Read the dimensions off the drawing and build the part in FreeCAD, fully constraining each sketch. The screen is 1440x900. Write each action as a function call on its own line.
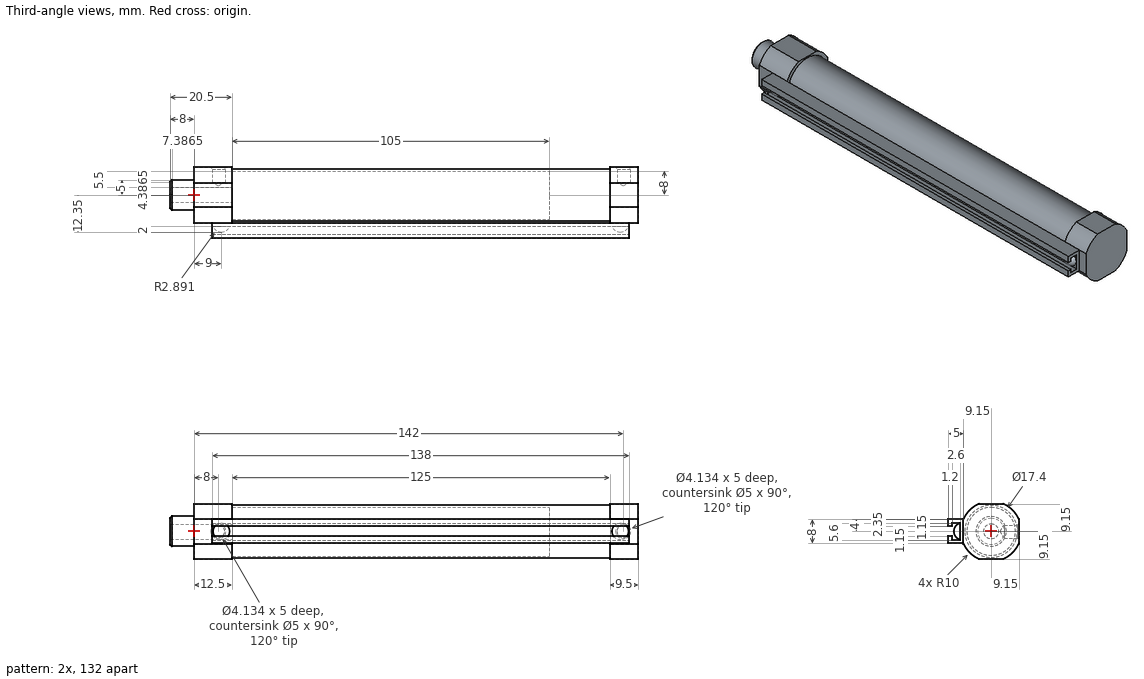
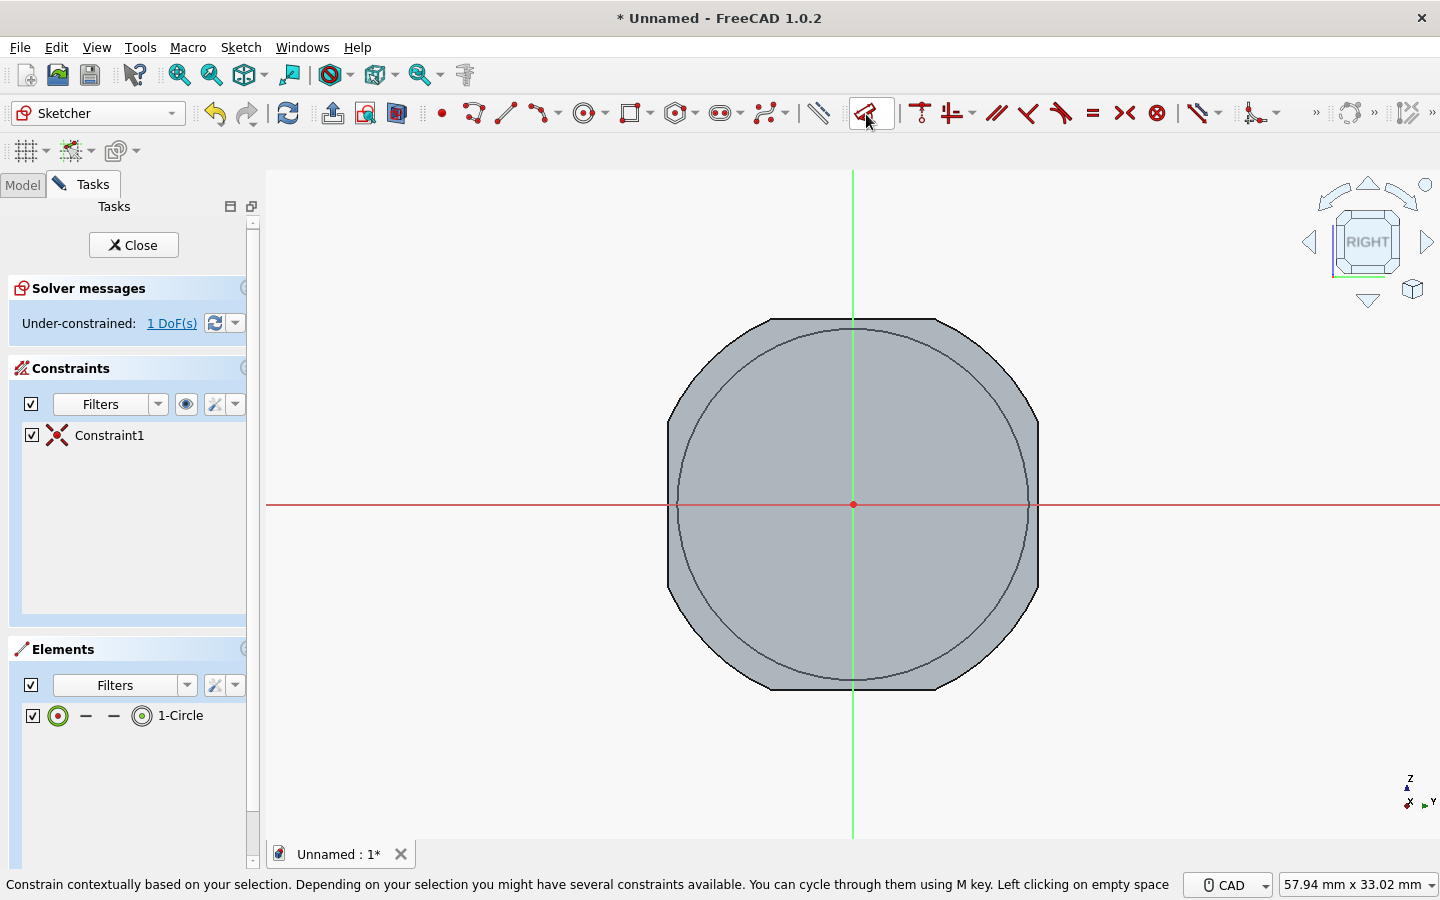
click(977, 380)
click(1000, 357)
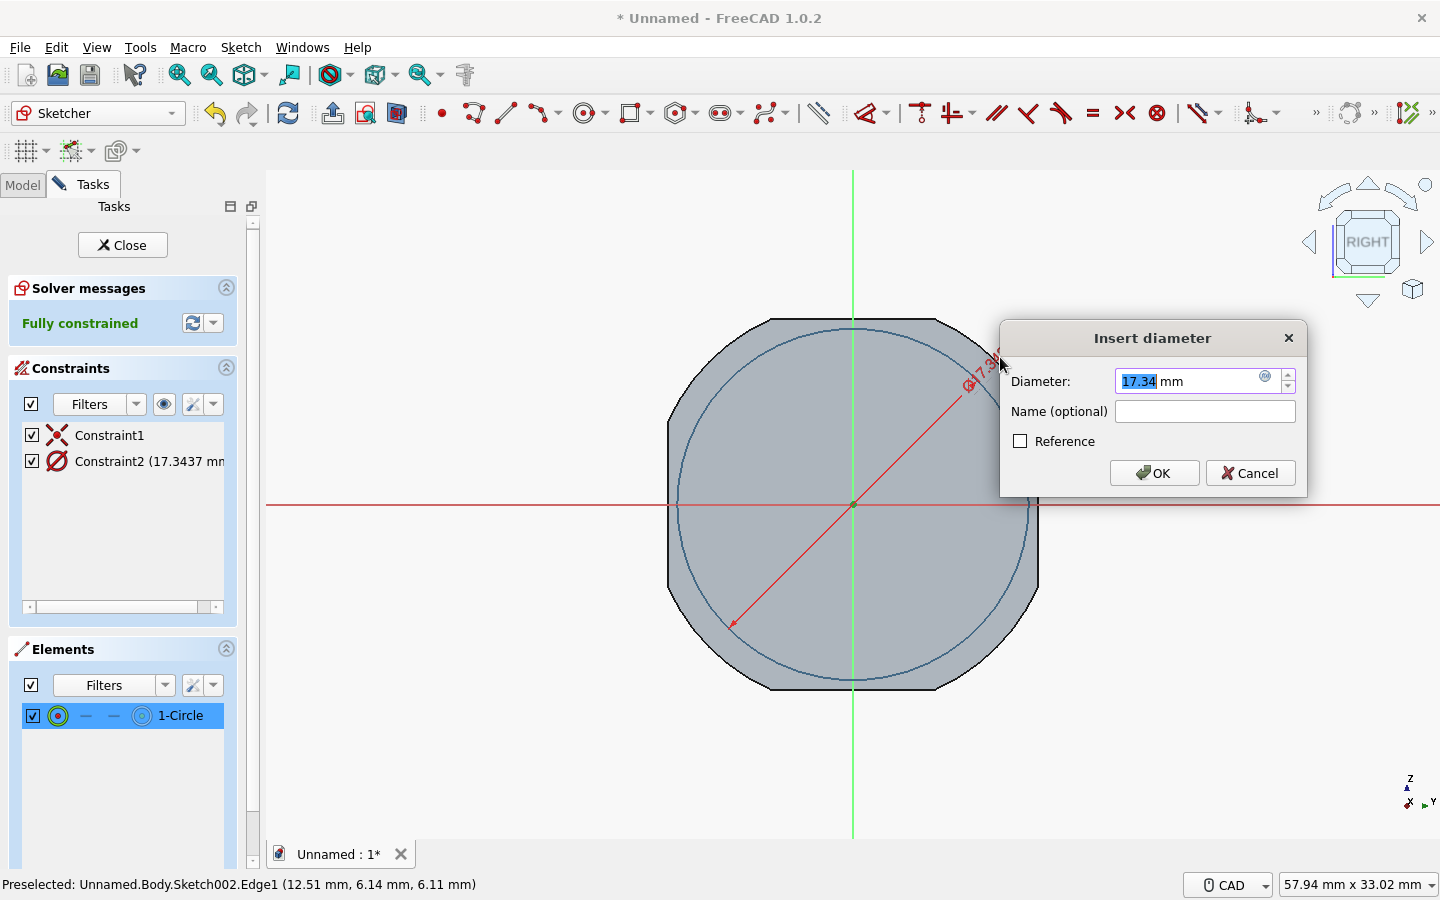
text(17.4)
key(Return)
key(Escape)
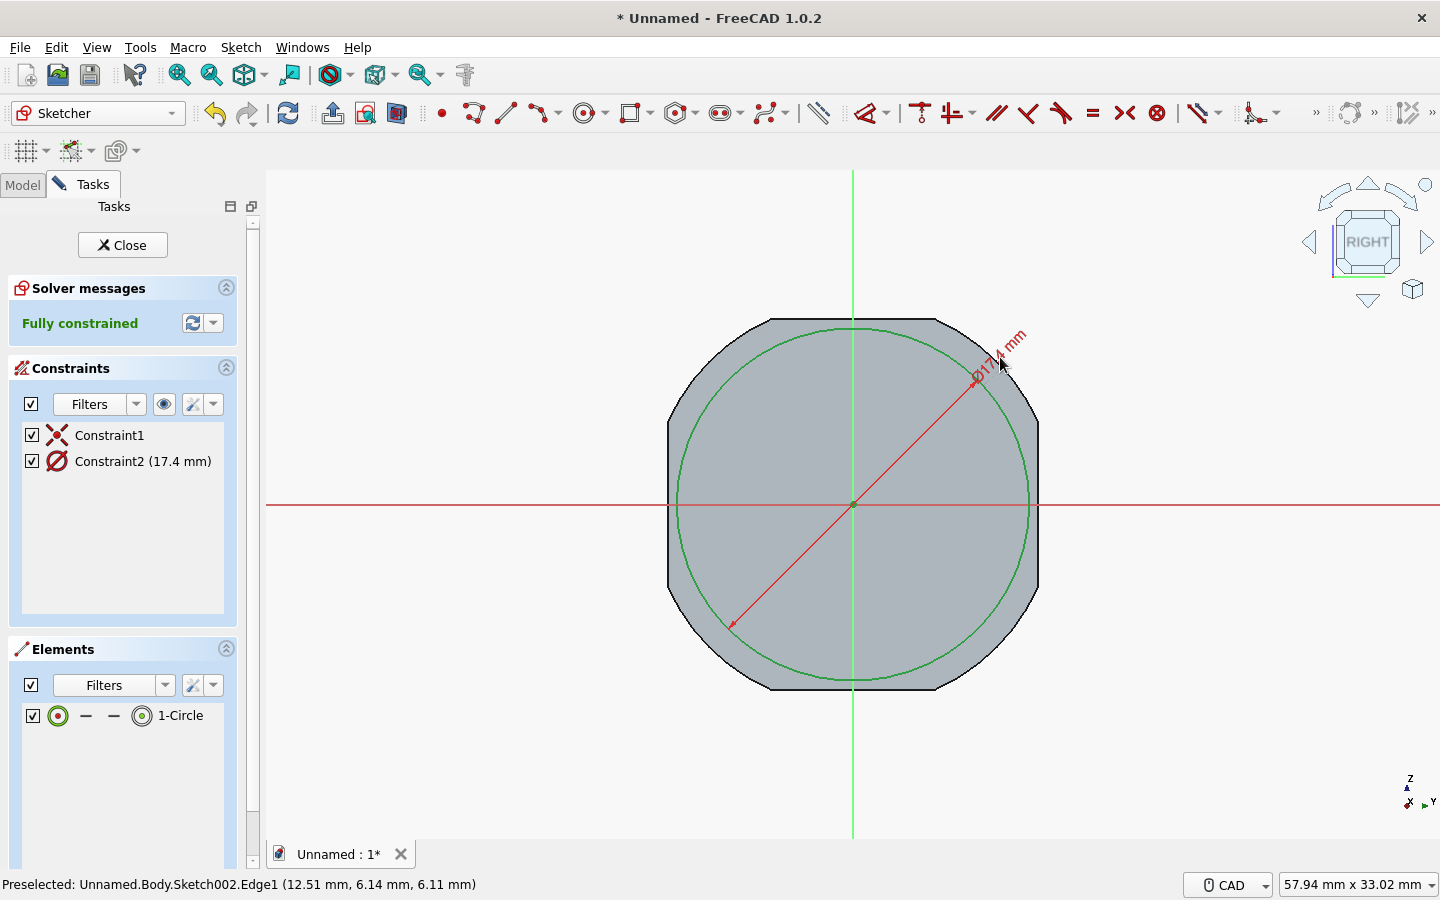
click(123, 245)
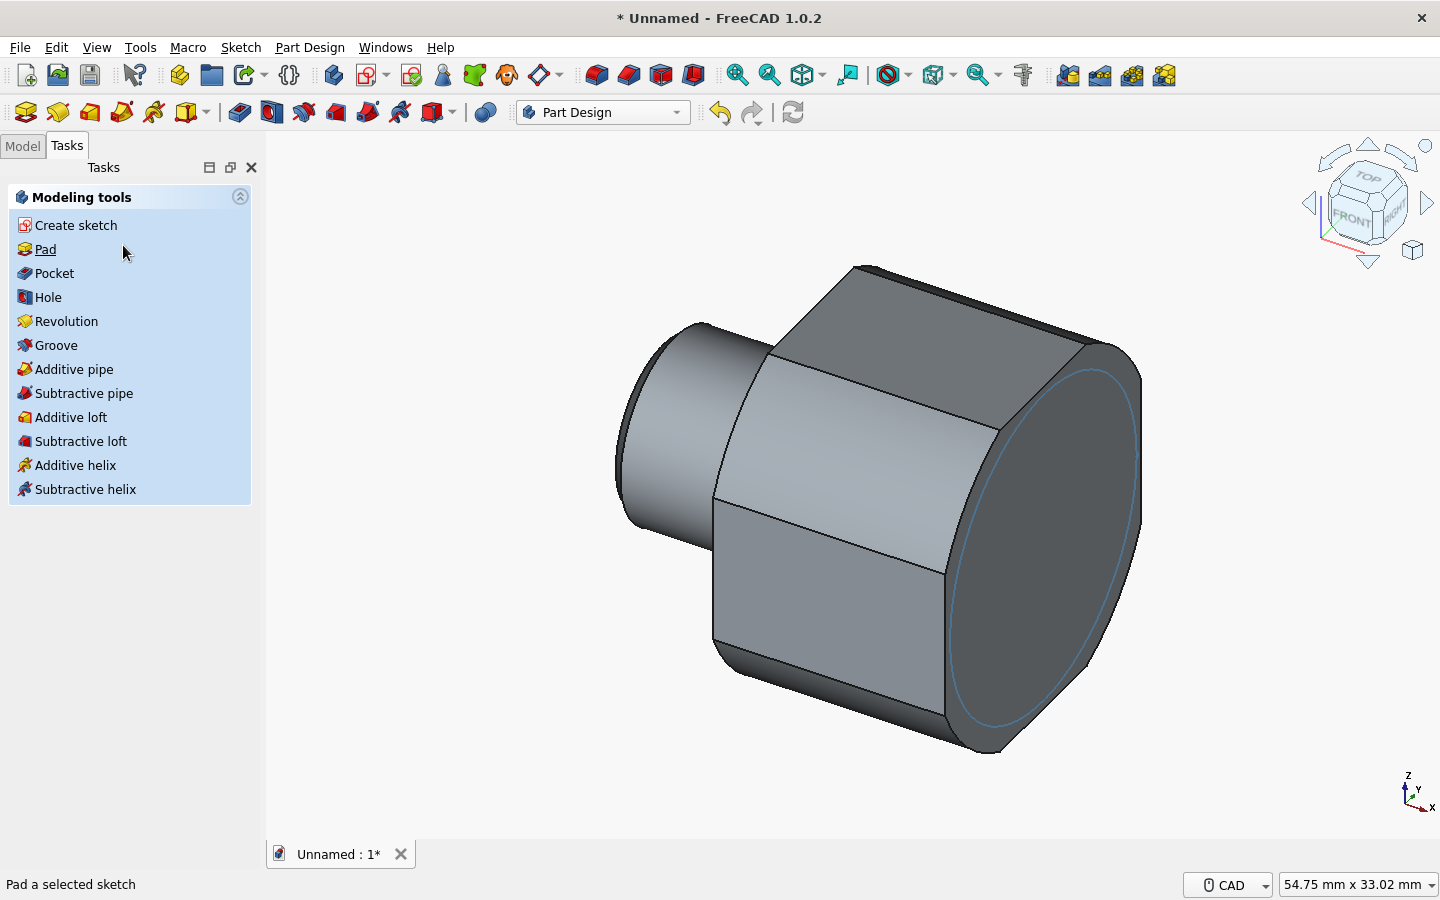
click(26, 112)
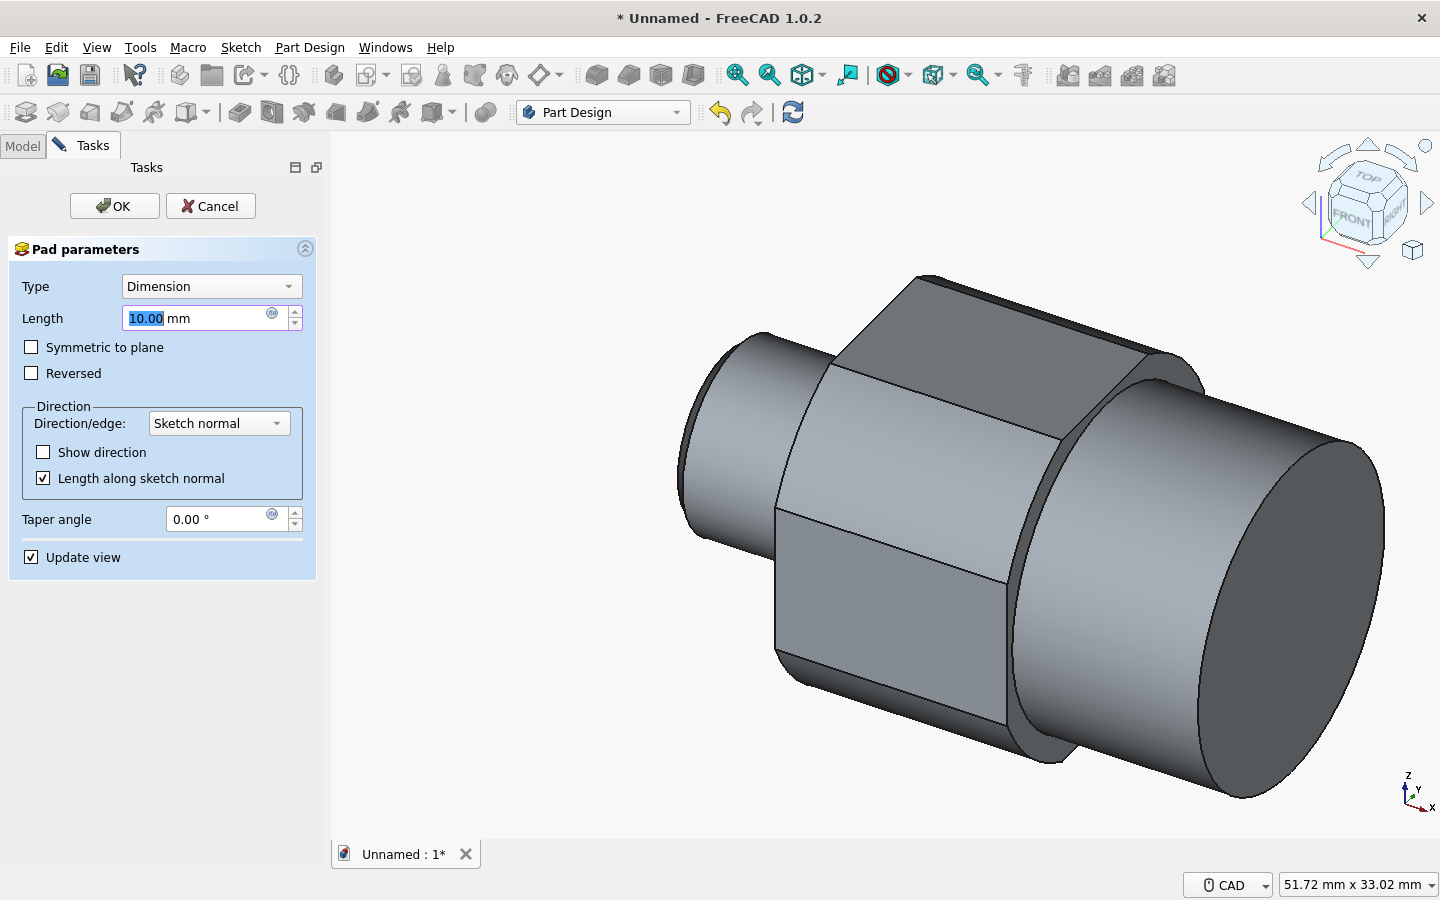
text(125)
key(Tab)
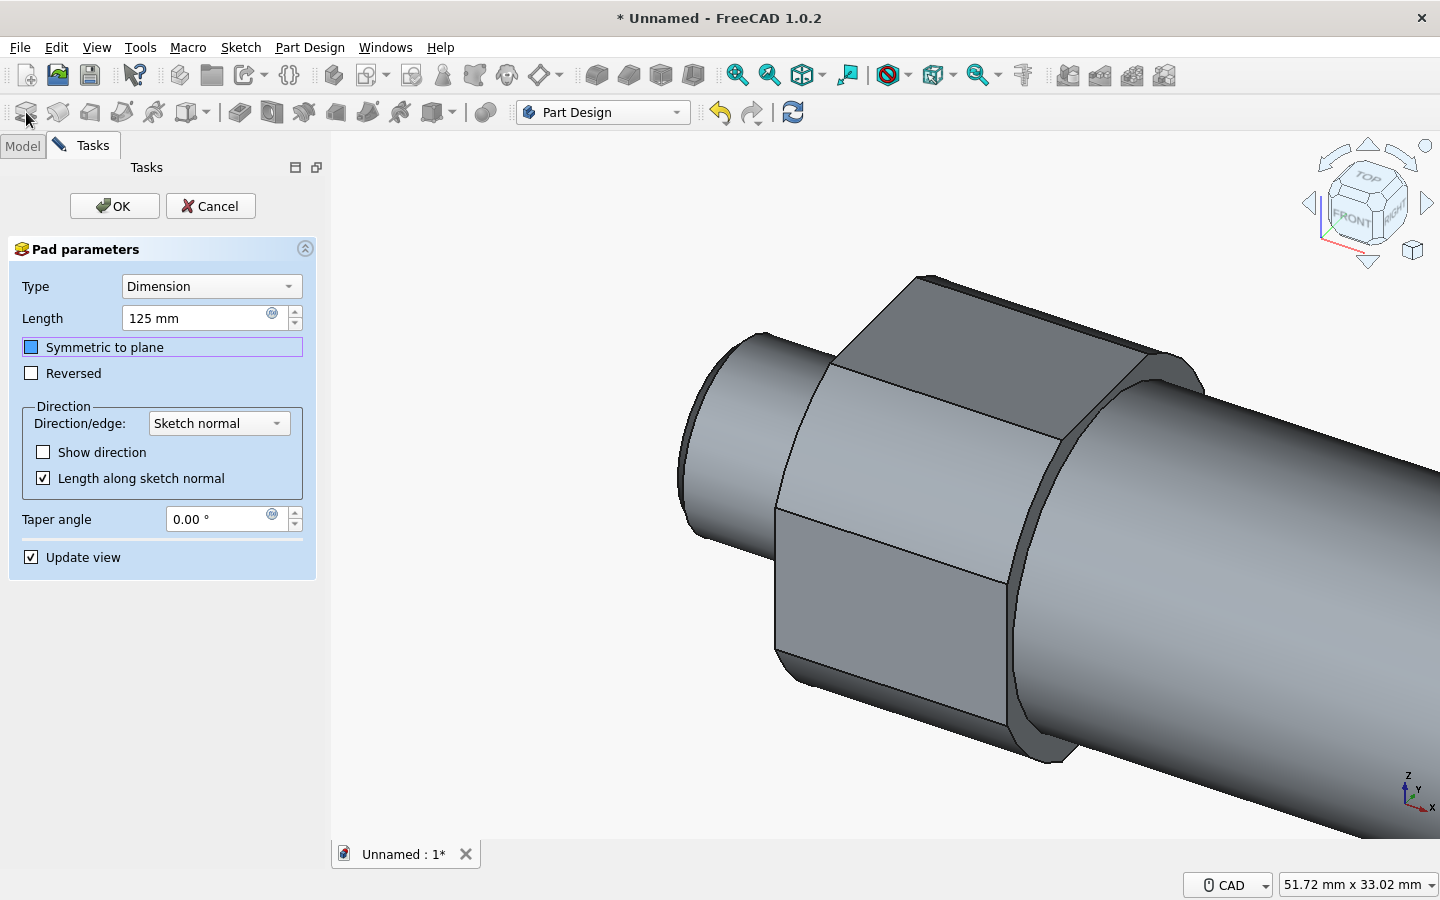
click(115, 206)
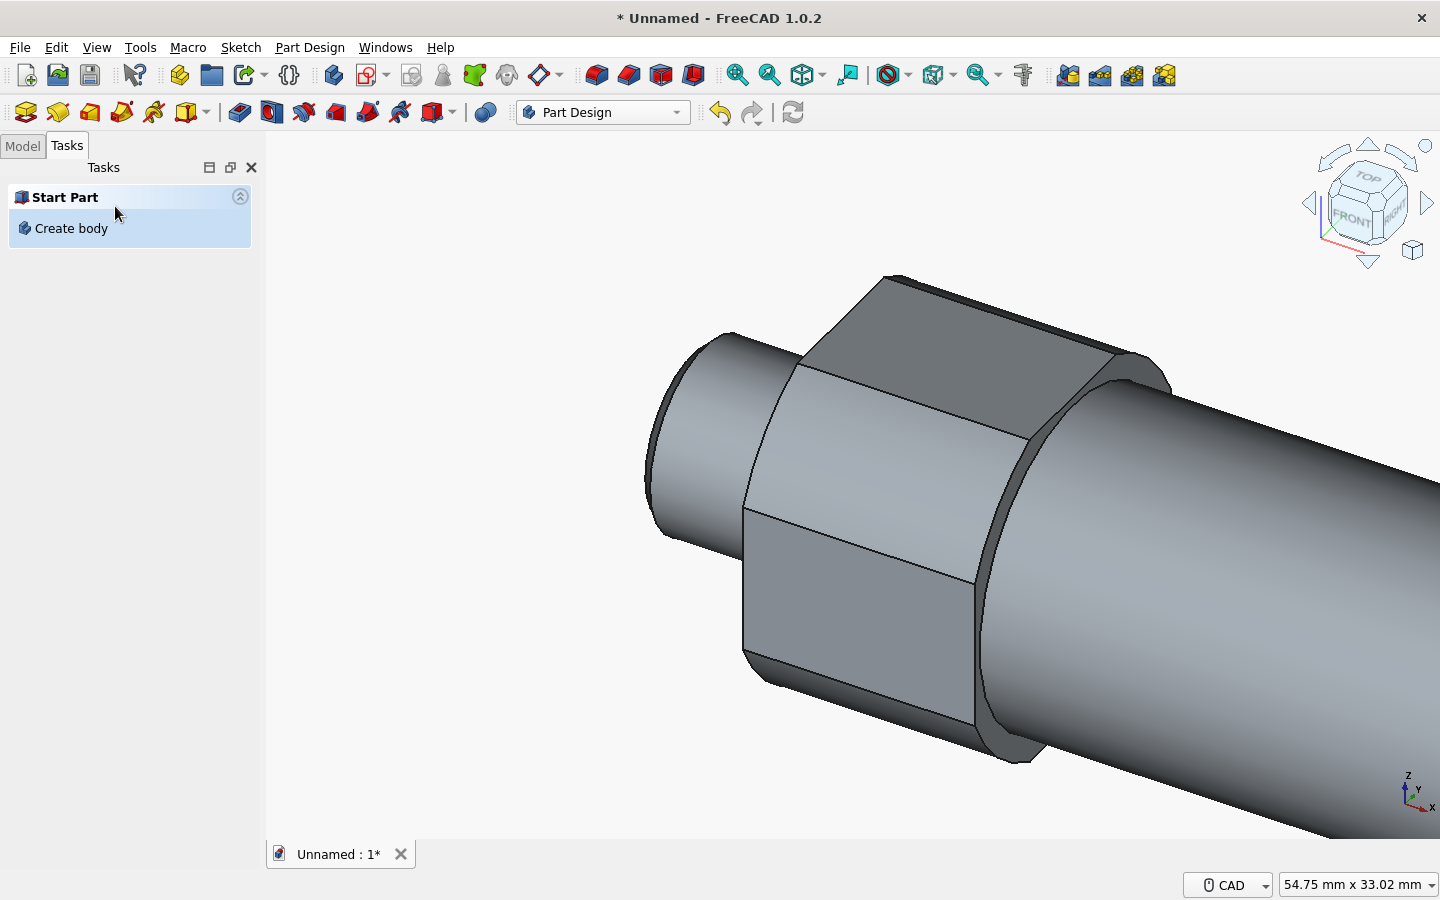
click(738, 76)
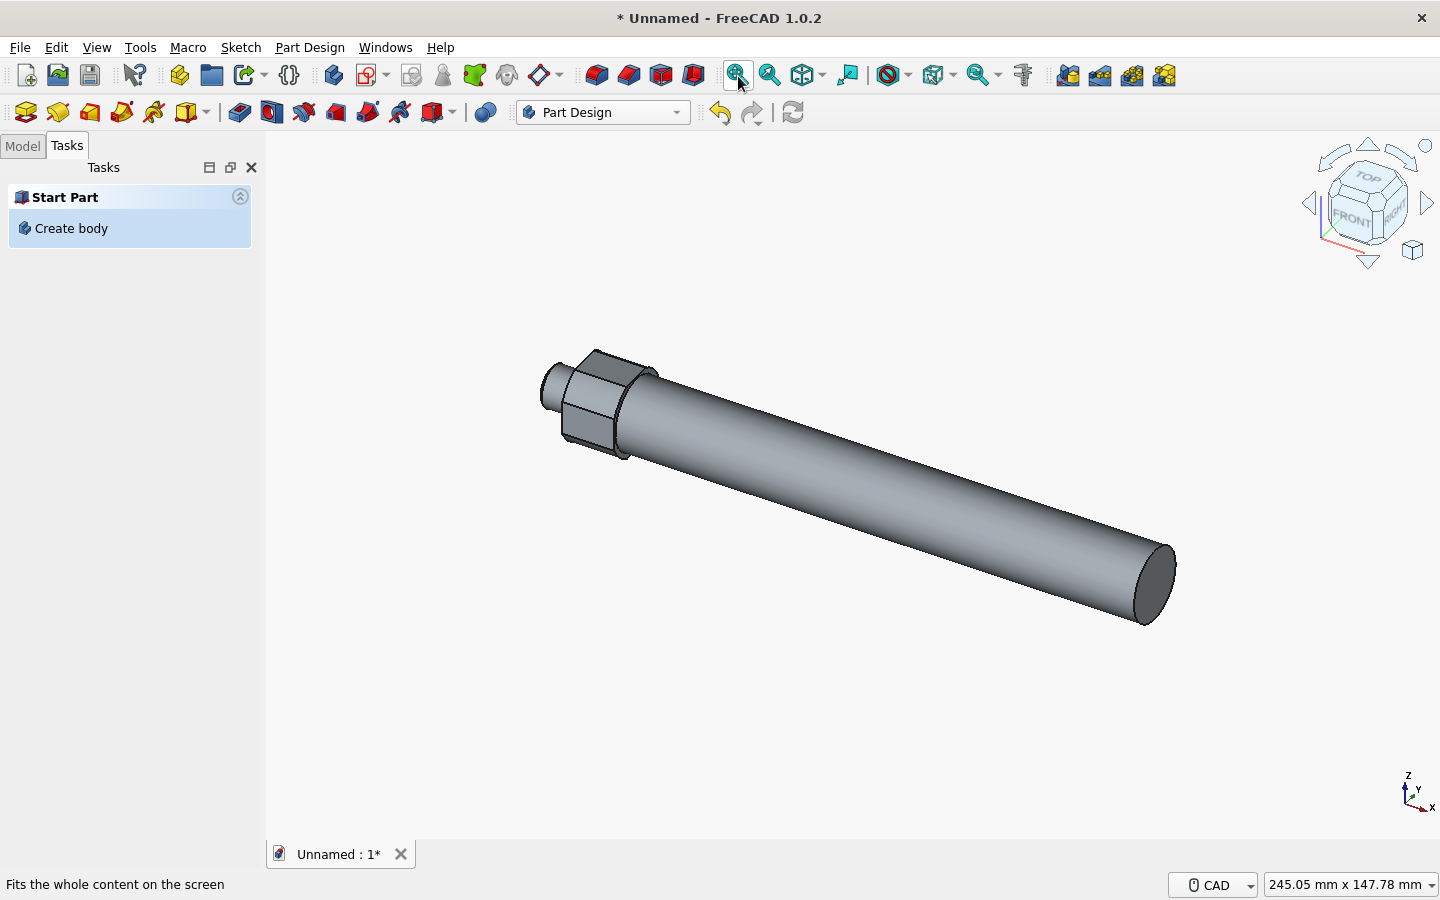
click(1155, 584)